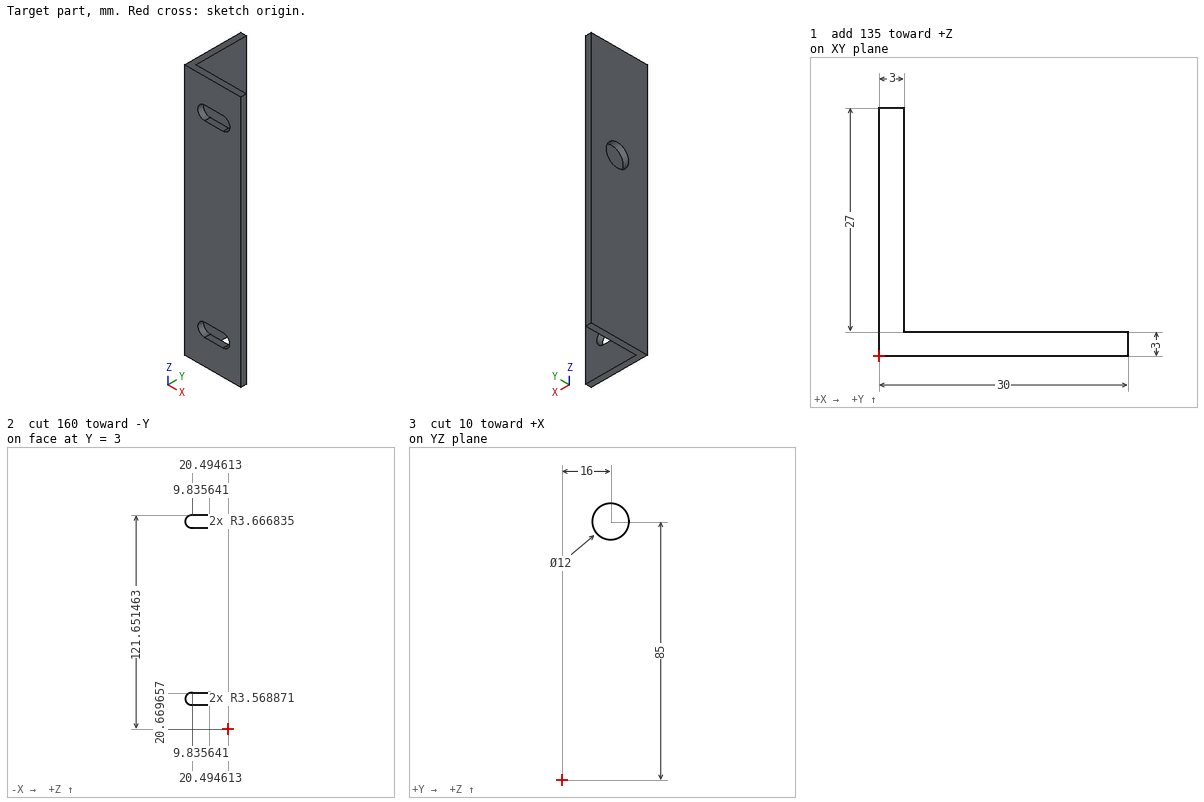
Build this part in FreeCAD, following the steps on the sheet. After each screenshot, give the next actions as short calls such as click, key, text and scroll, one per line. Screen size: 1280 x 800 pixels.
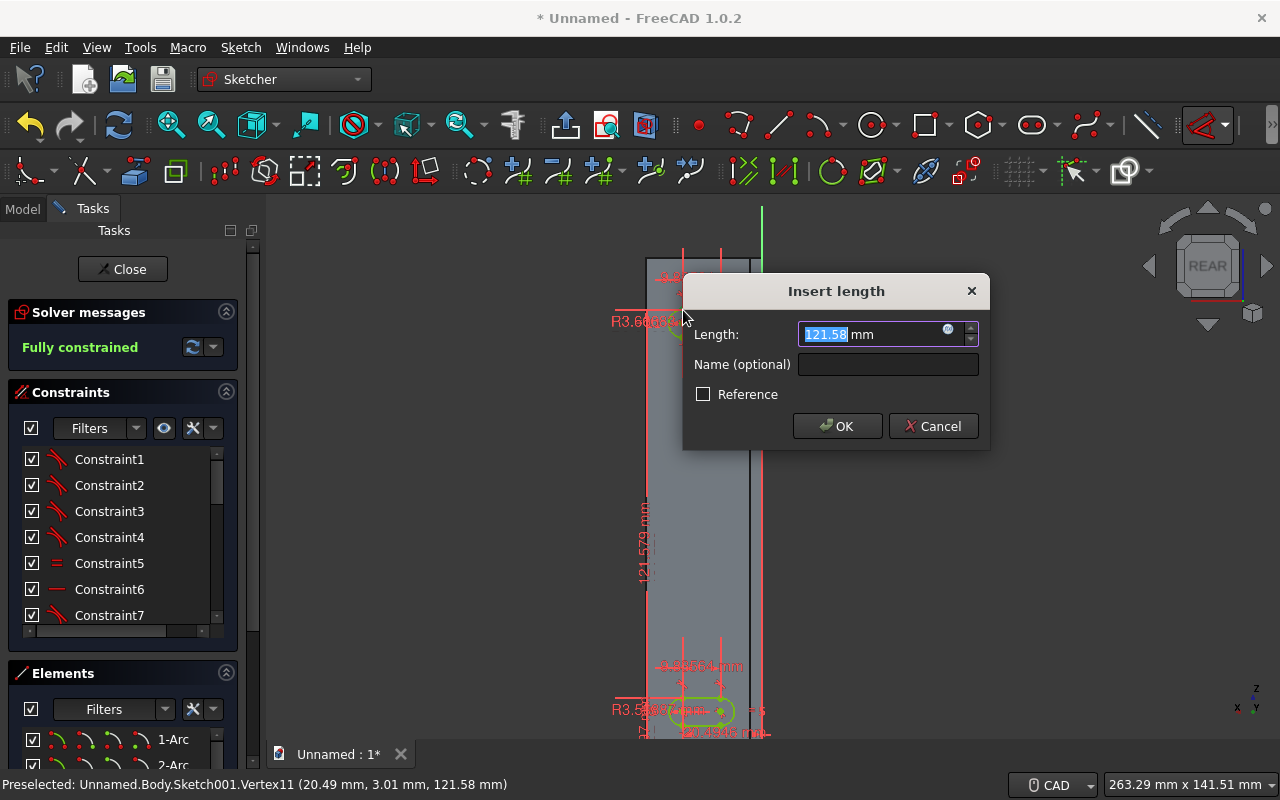
text(121.651463)
key(Return)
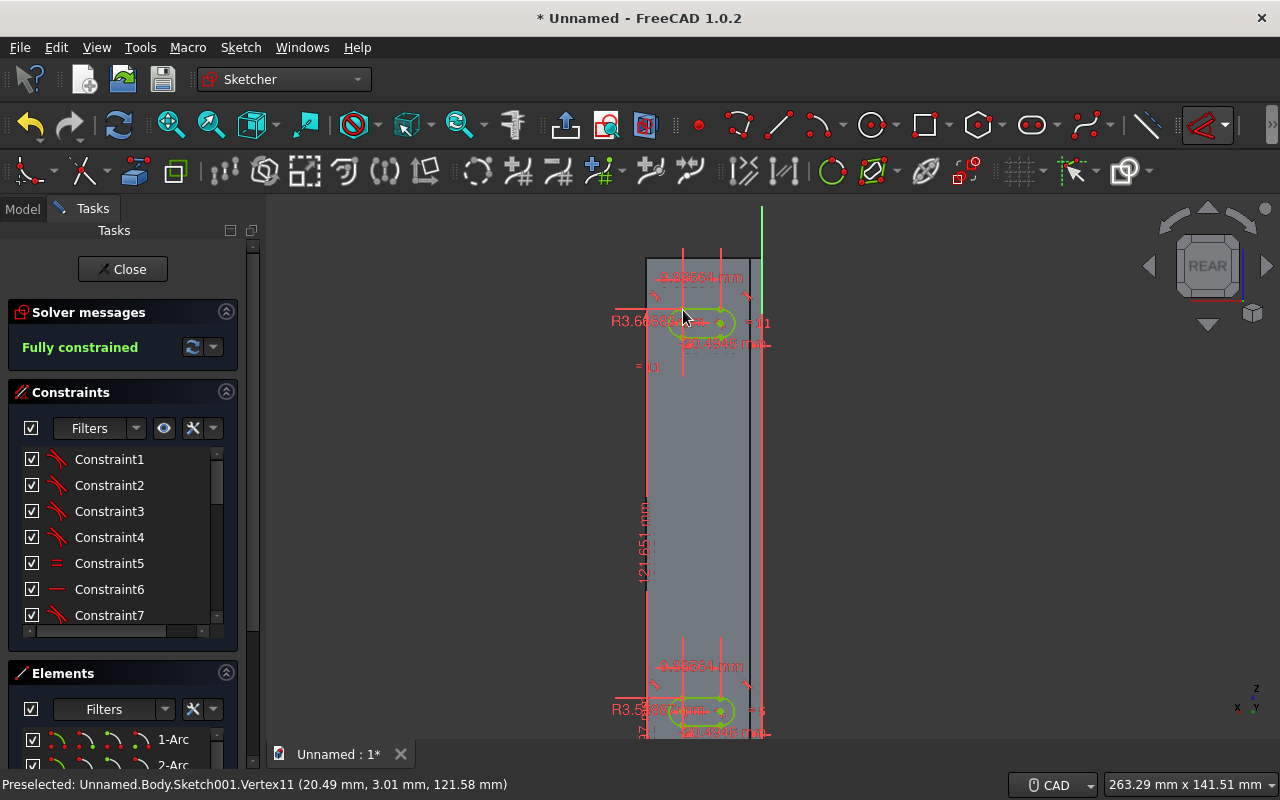
click(123, 269)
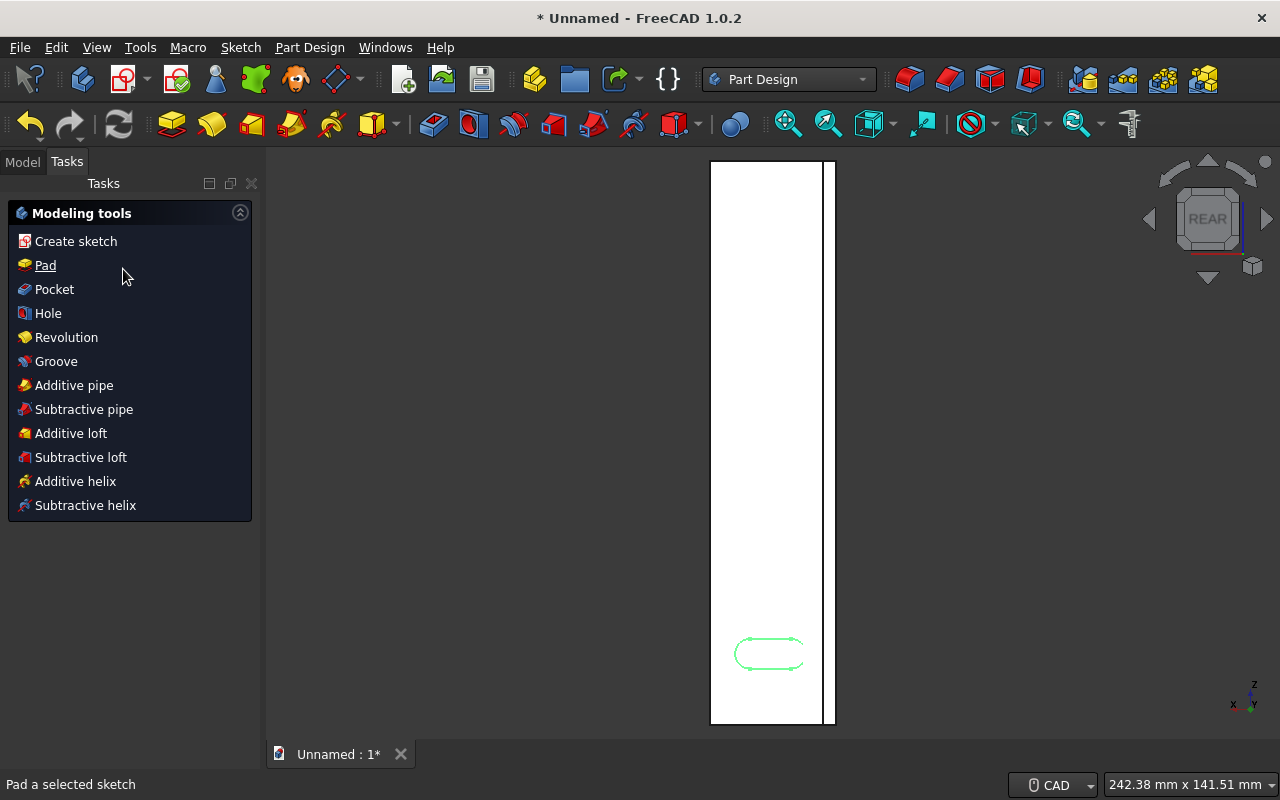
click(434, 124)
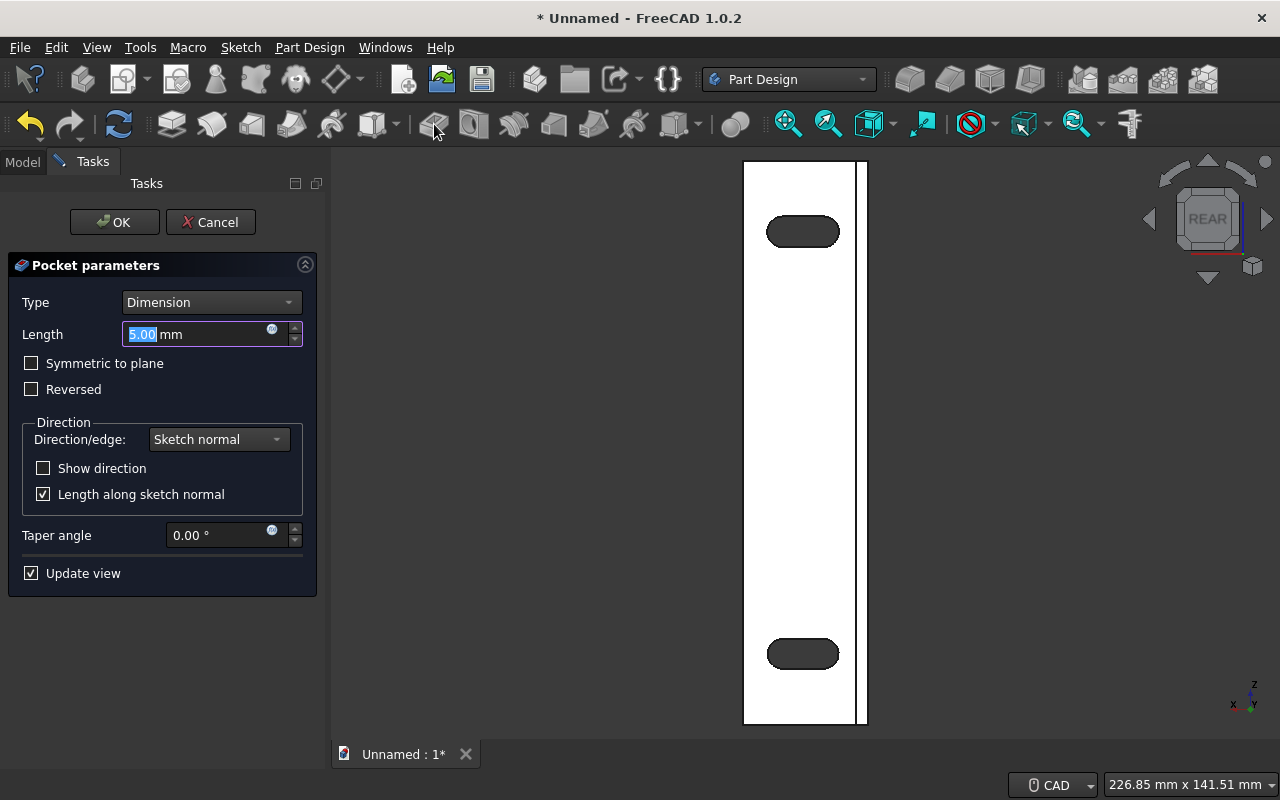
text(160)
key(Tab)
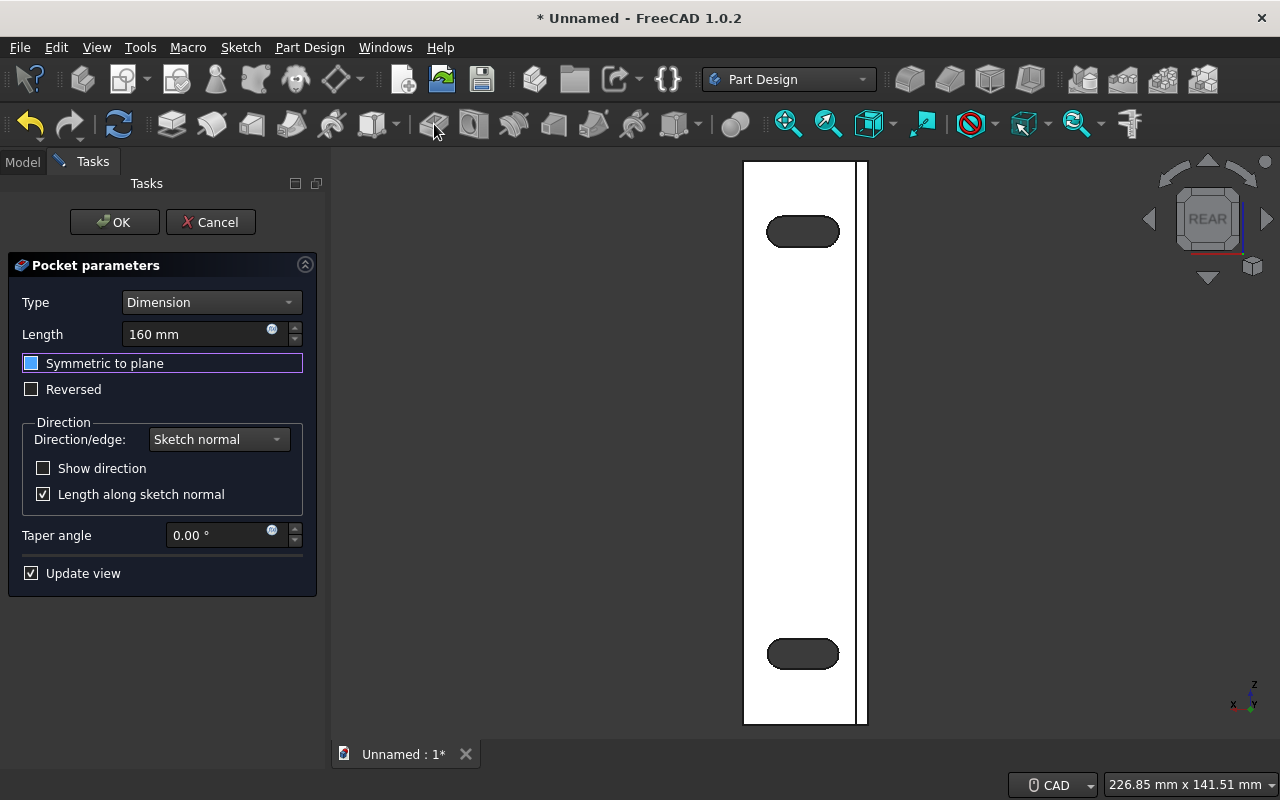
click(115, 222)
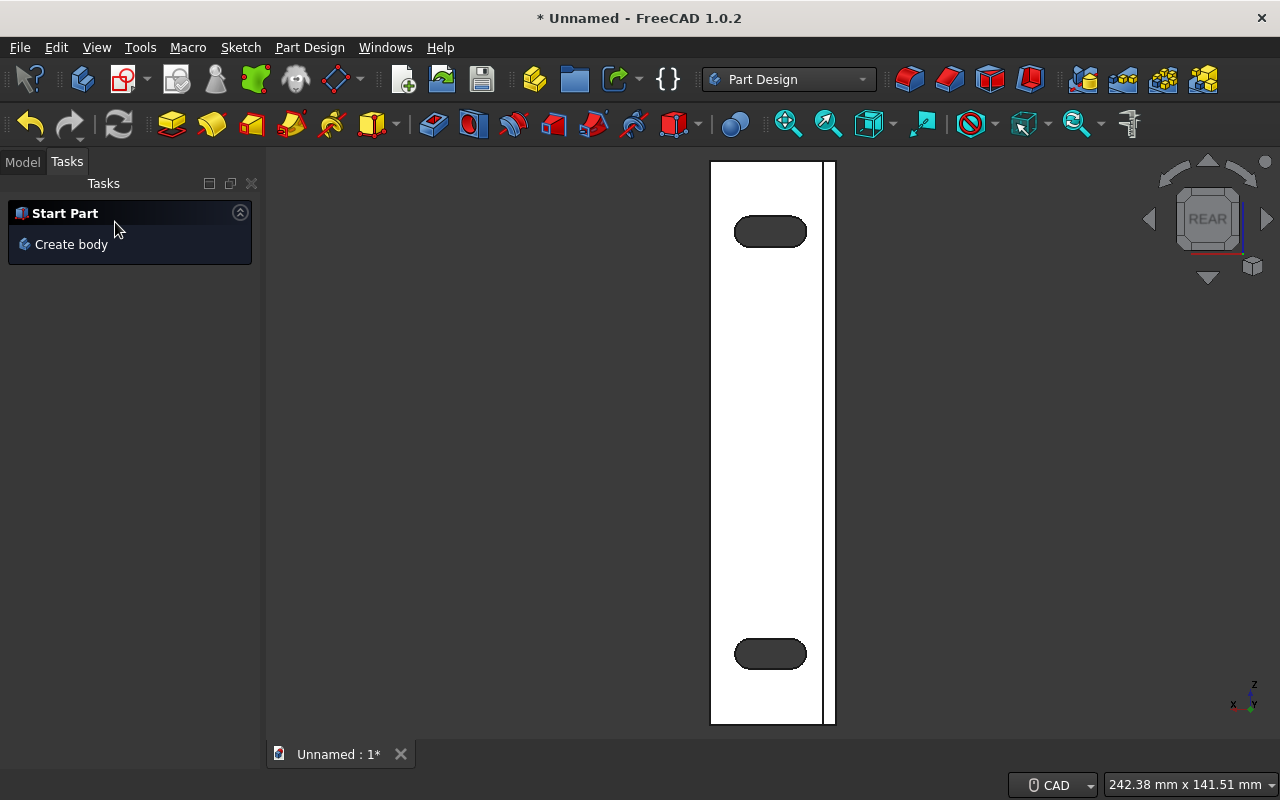
click(124, 80)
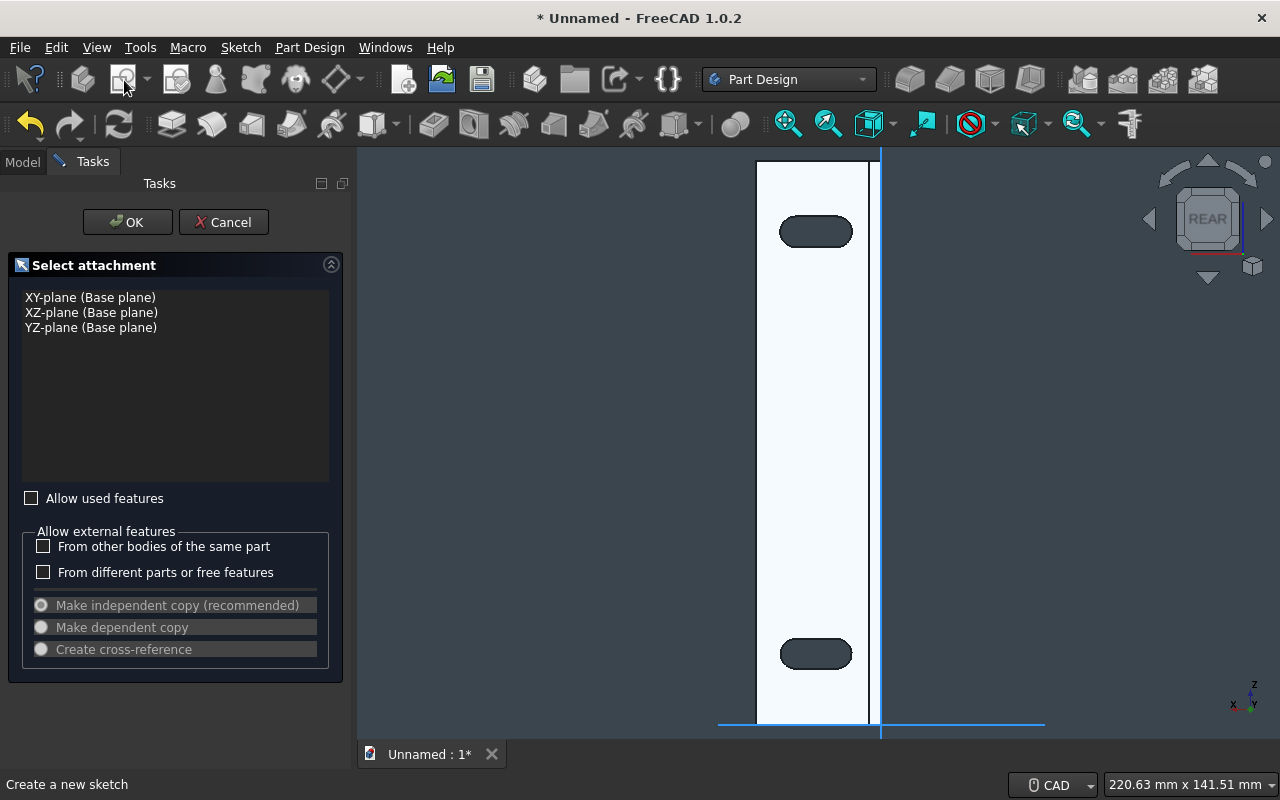
click(82, 328)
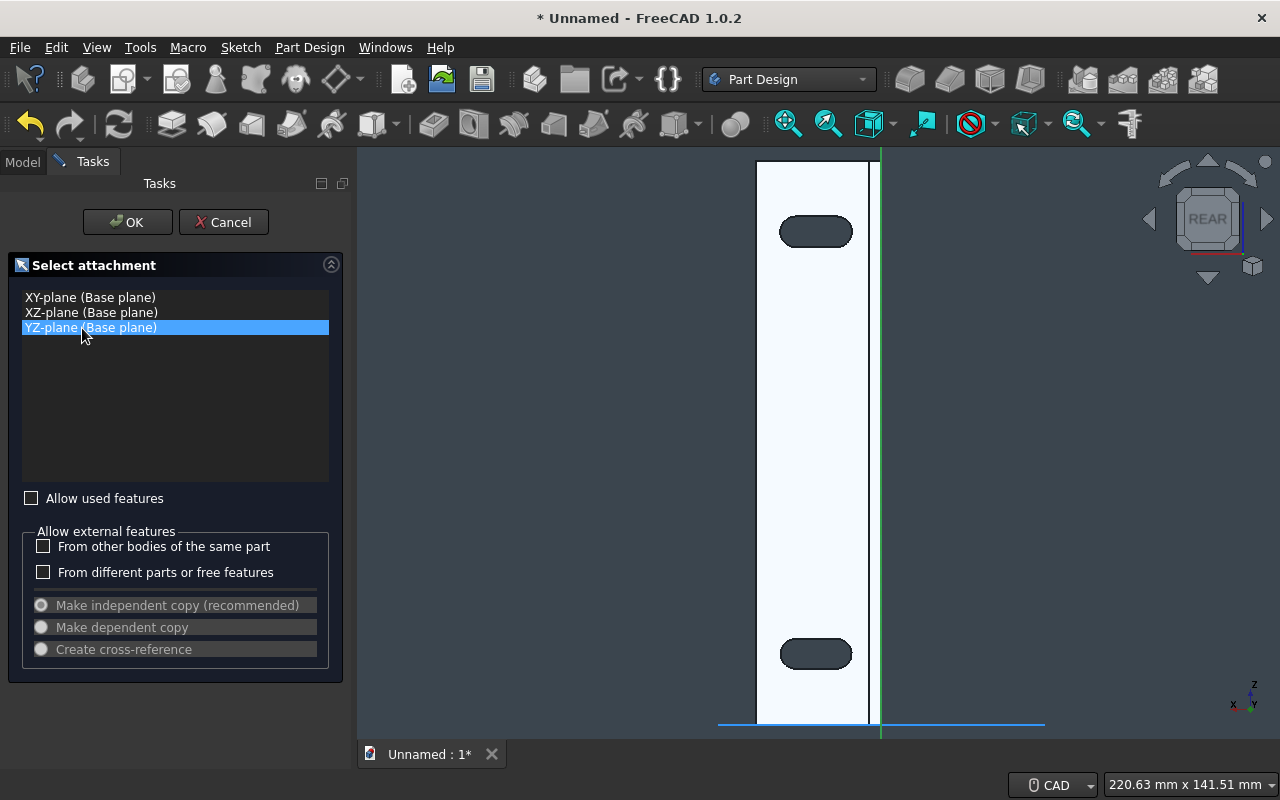
click(128, 222)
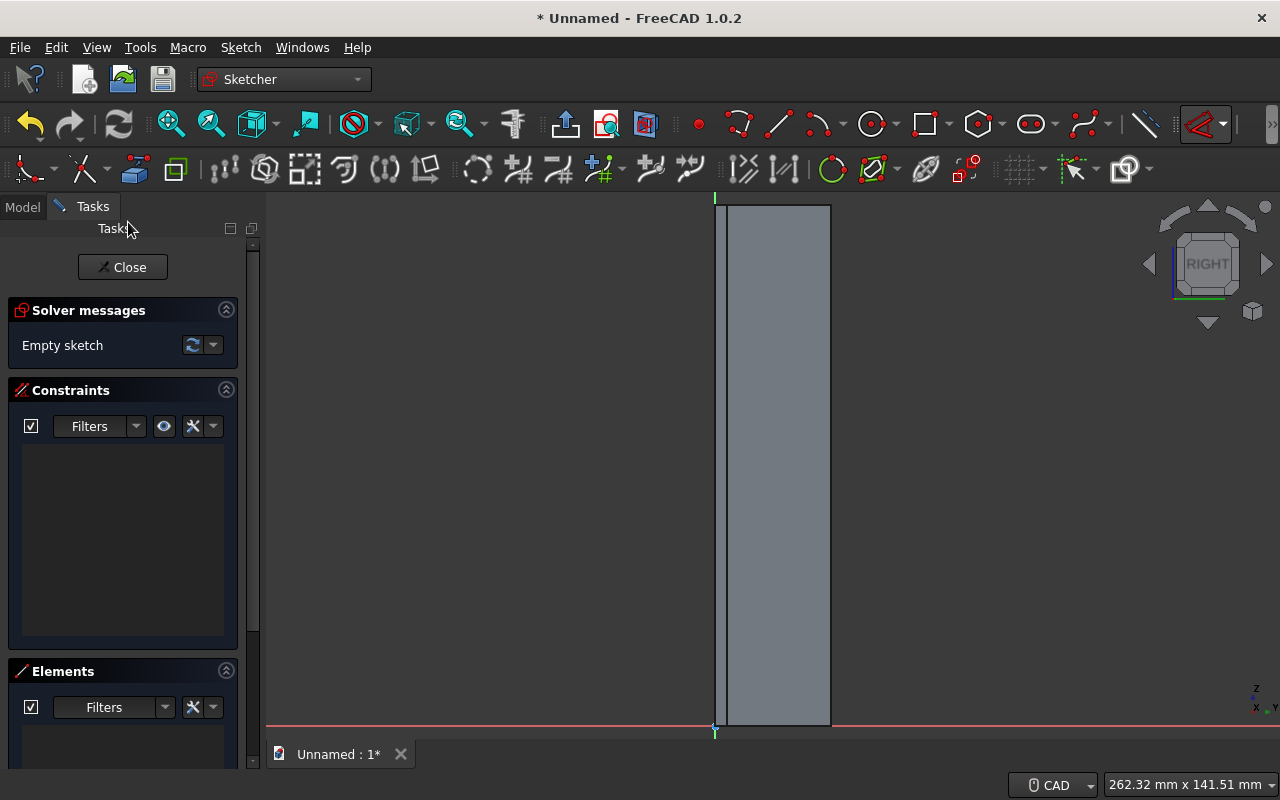
key(q)
key(s)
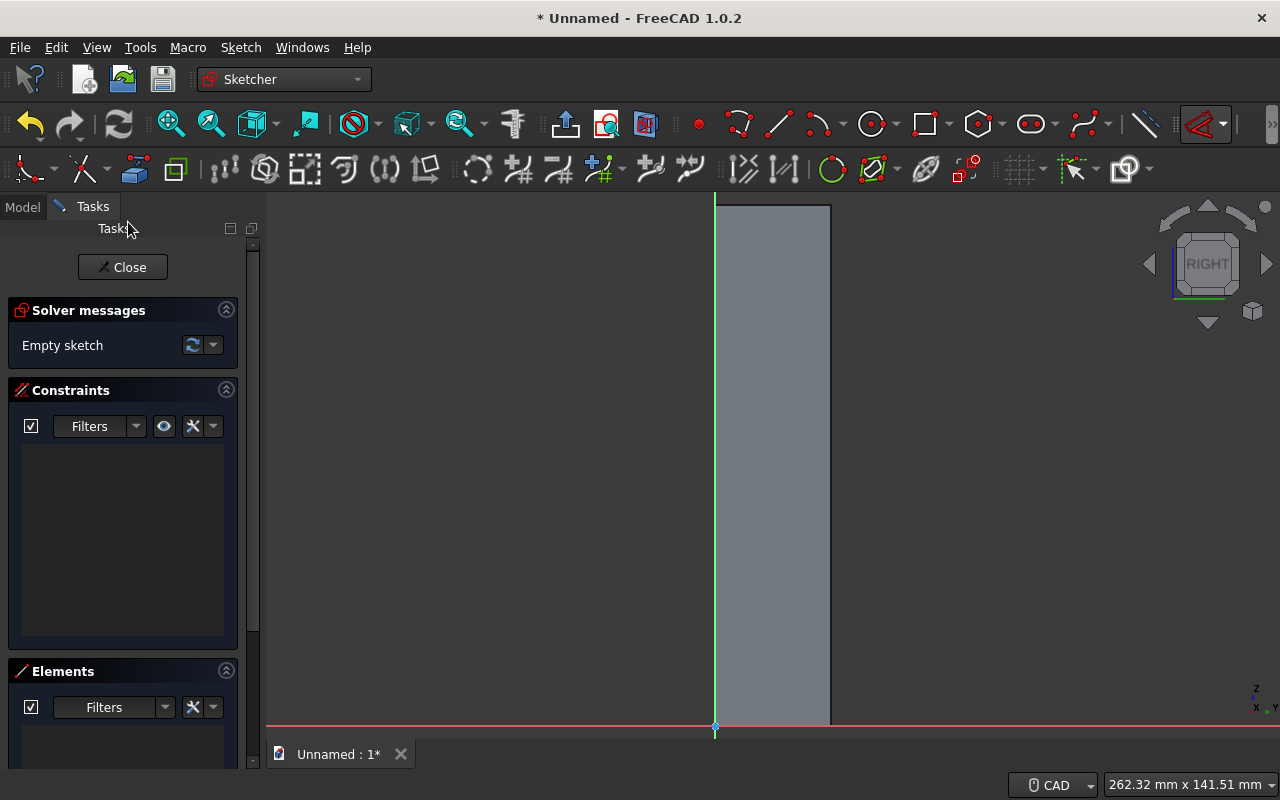
scroll(788, 387, up, 10)